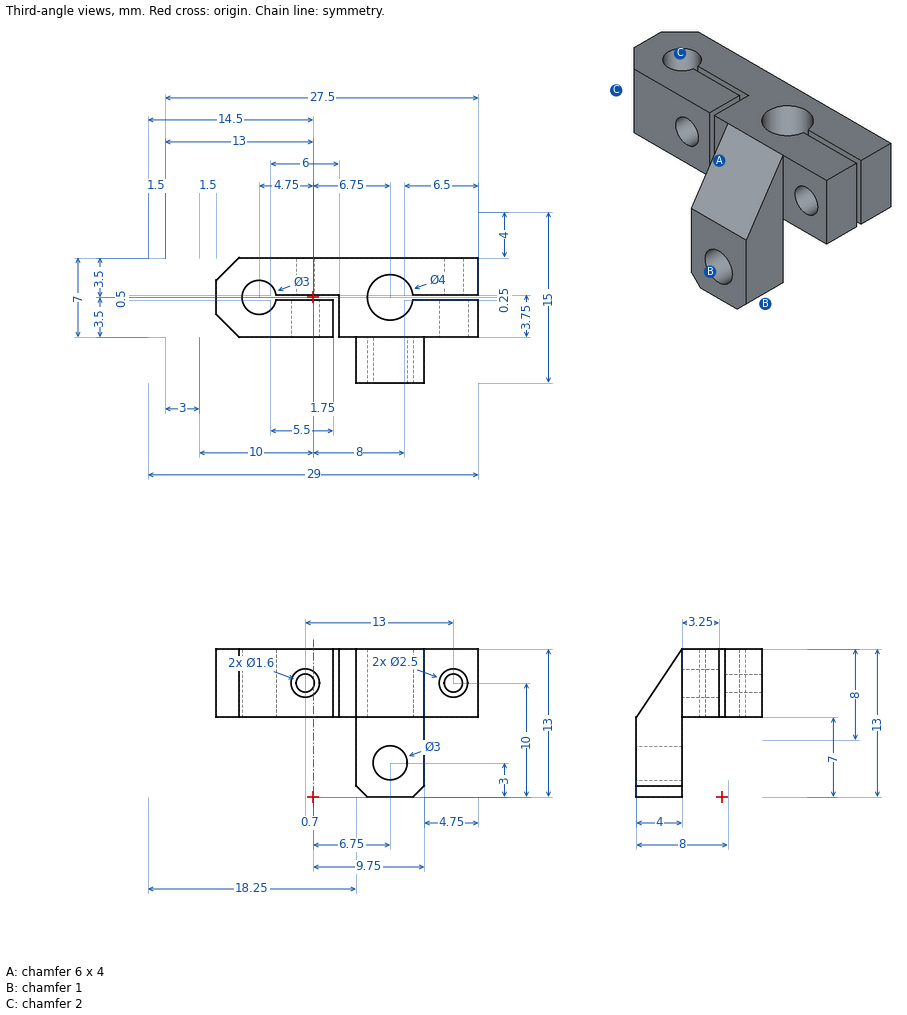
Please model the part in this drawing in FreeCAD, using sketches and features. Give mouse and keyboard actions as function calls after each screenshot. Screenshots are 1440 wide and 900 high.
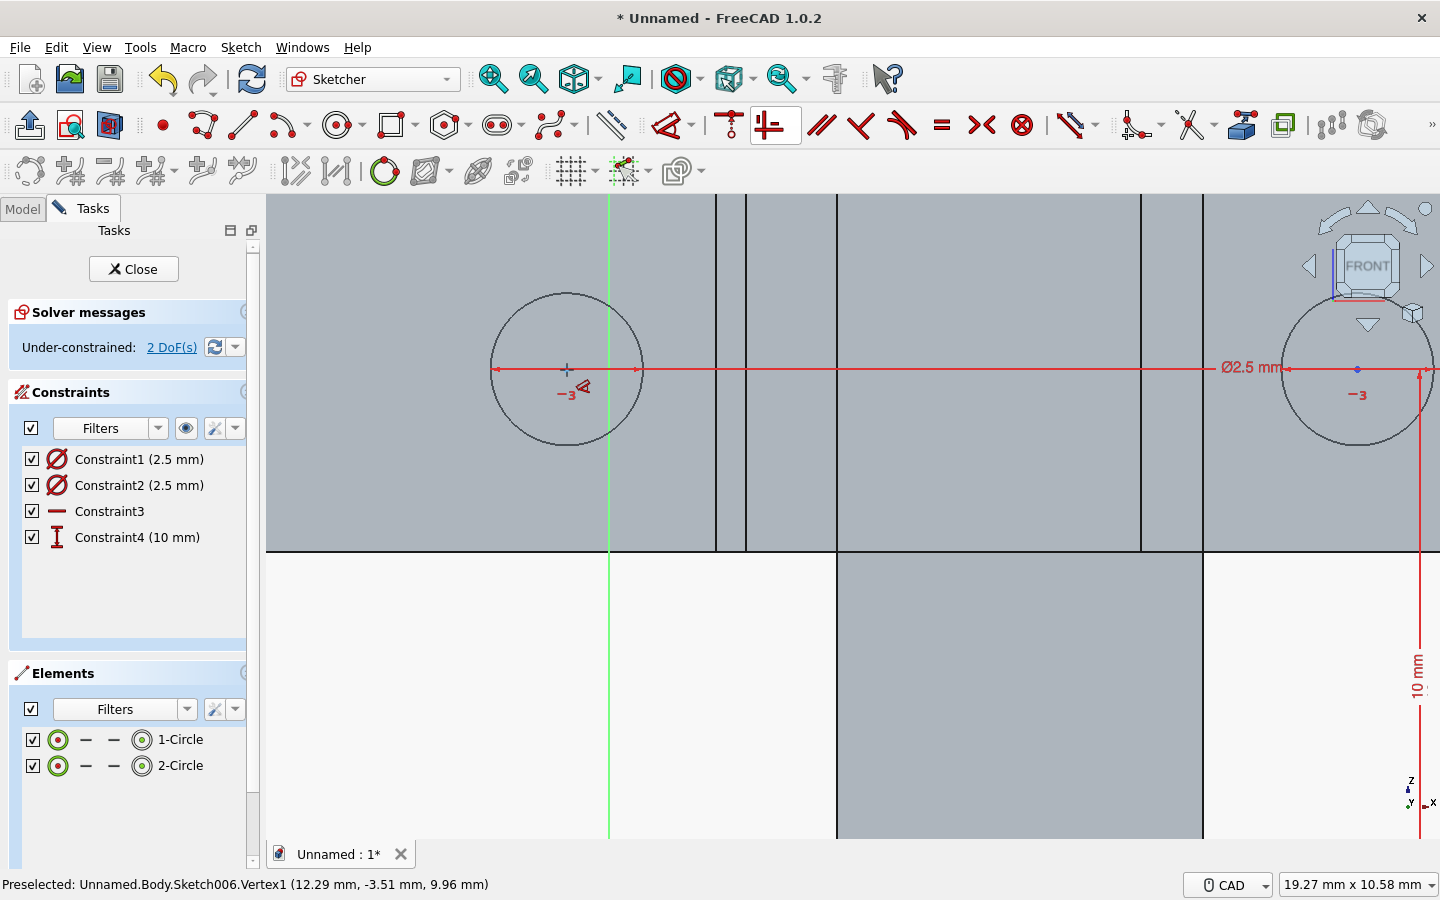
click(567, 369)
click(588, 335)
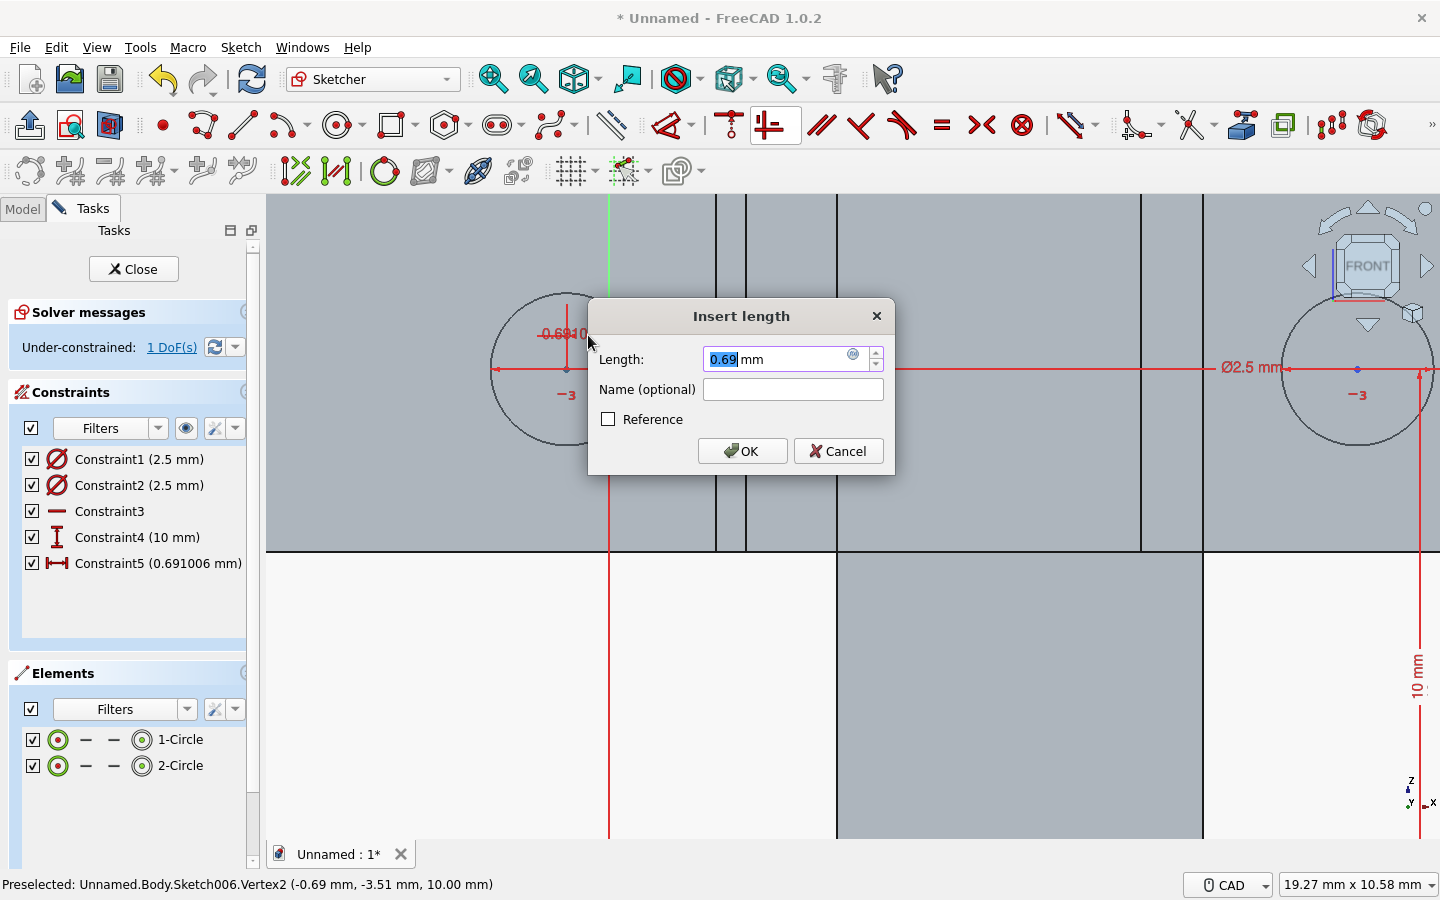
text(0.7)
key(Return)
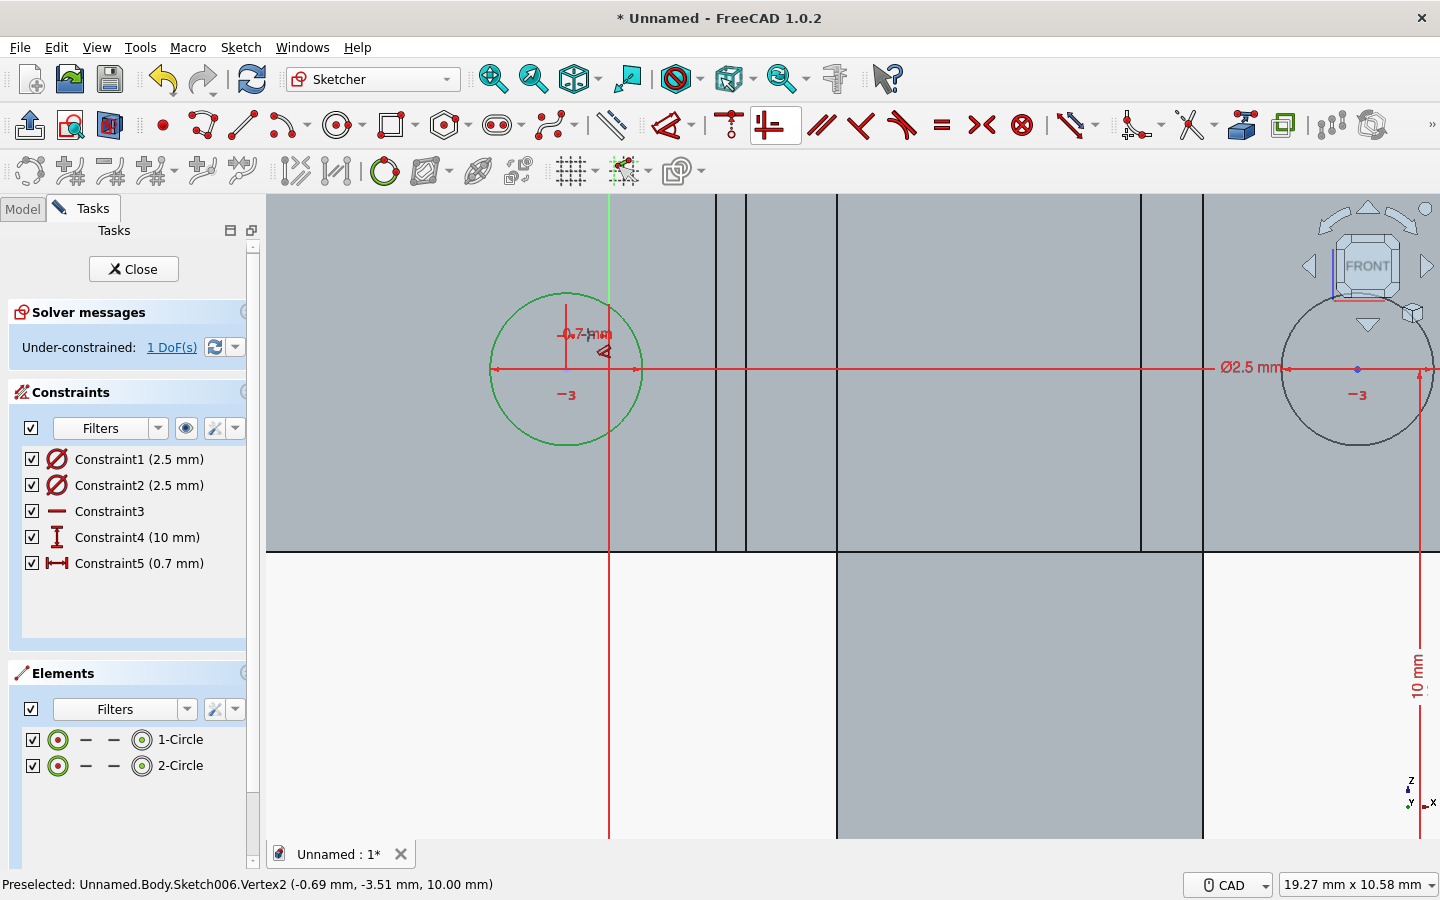
scroll(568, 371, down, 3)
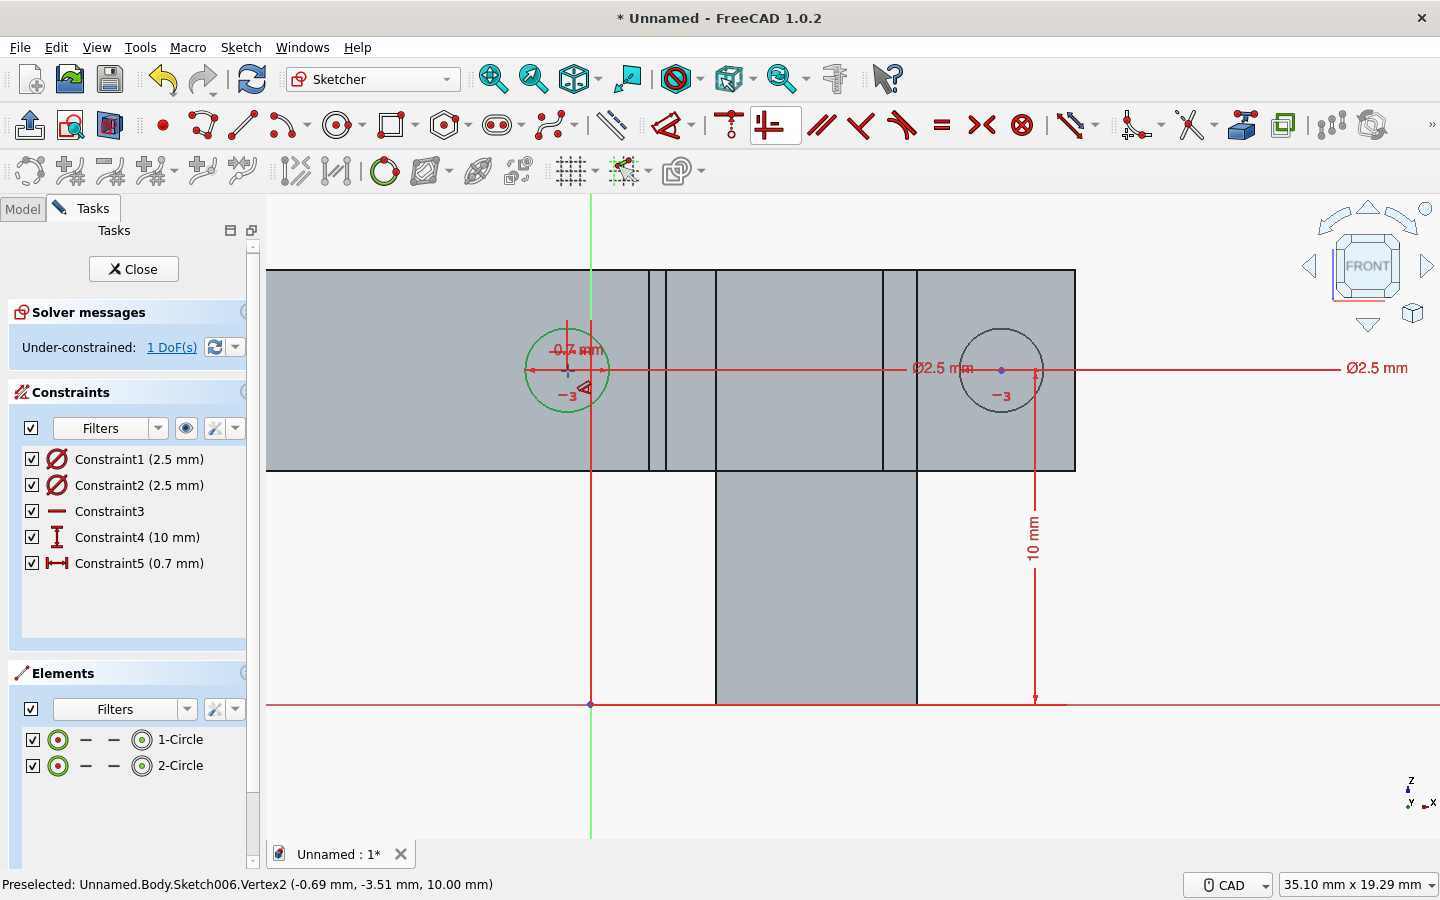
click(1001, 370)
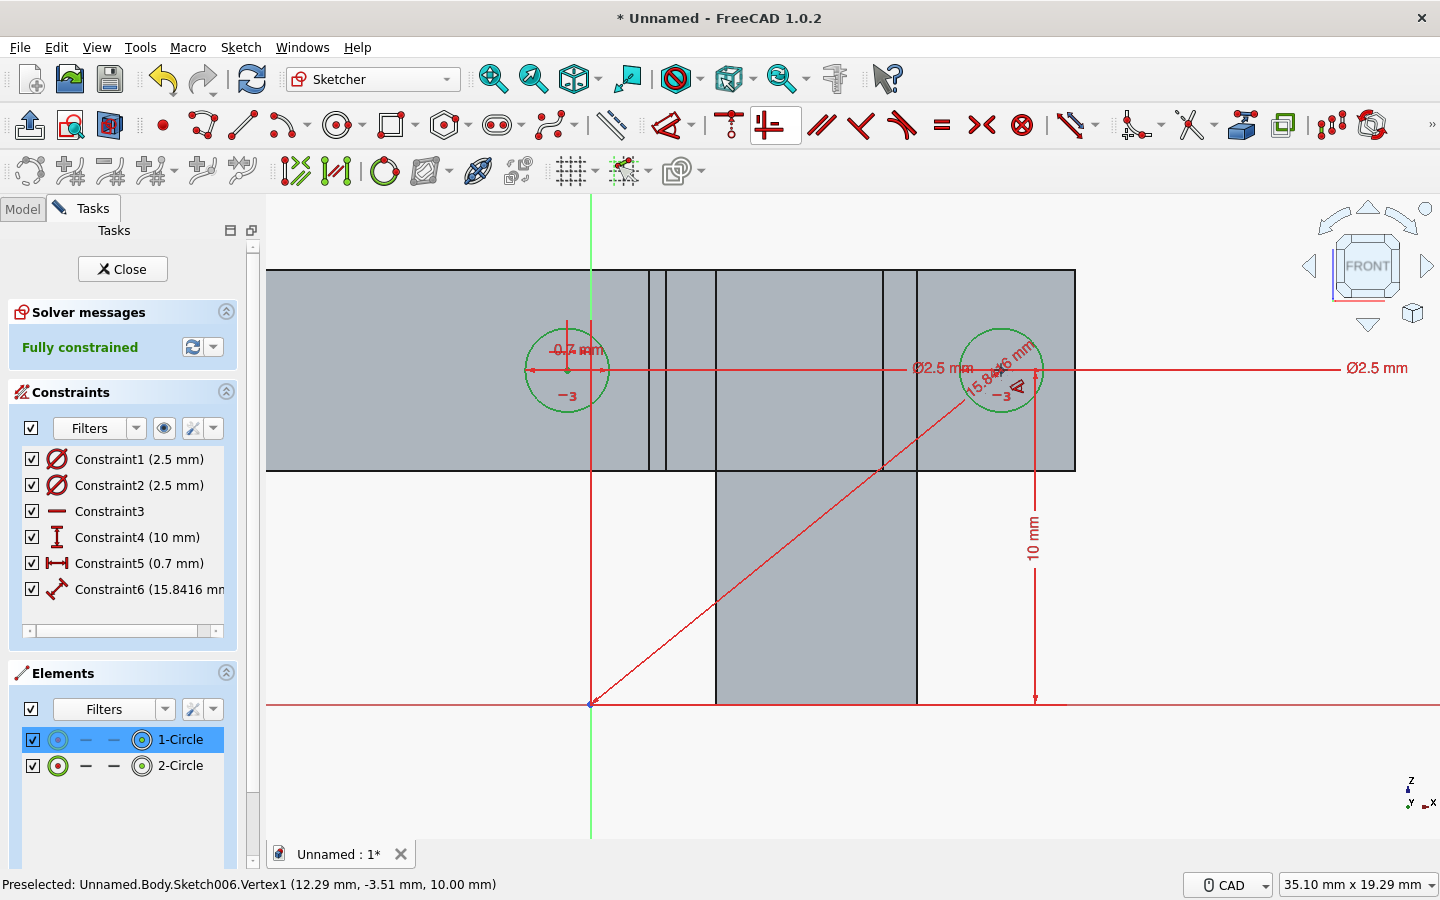
click(567, 370)
click(784, 336)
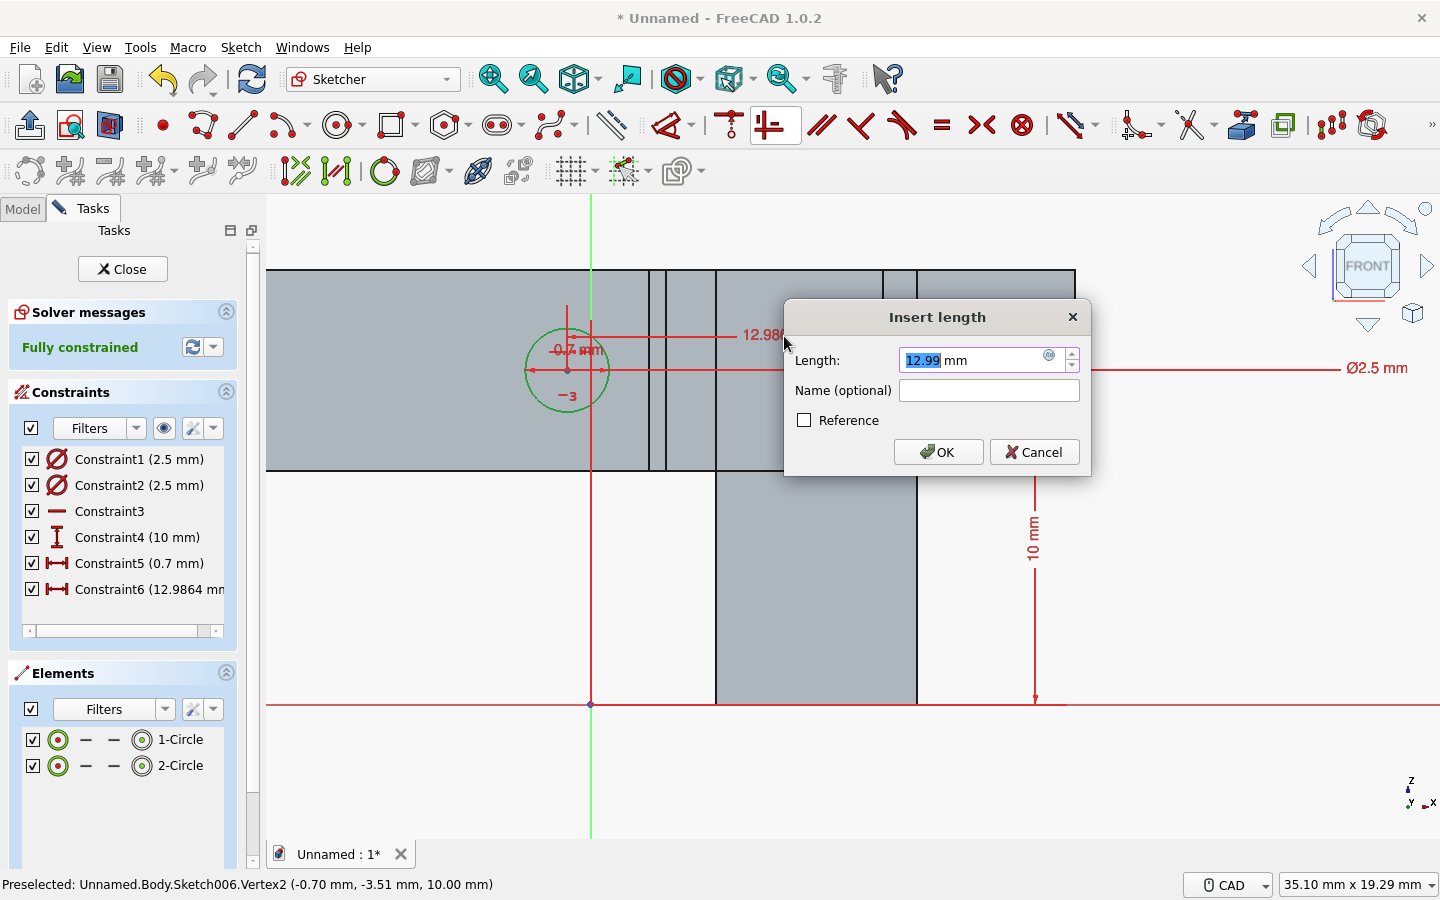
text(13)
key(Return)
key(Escape)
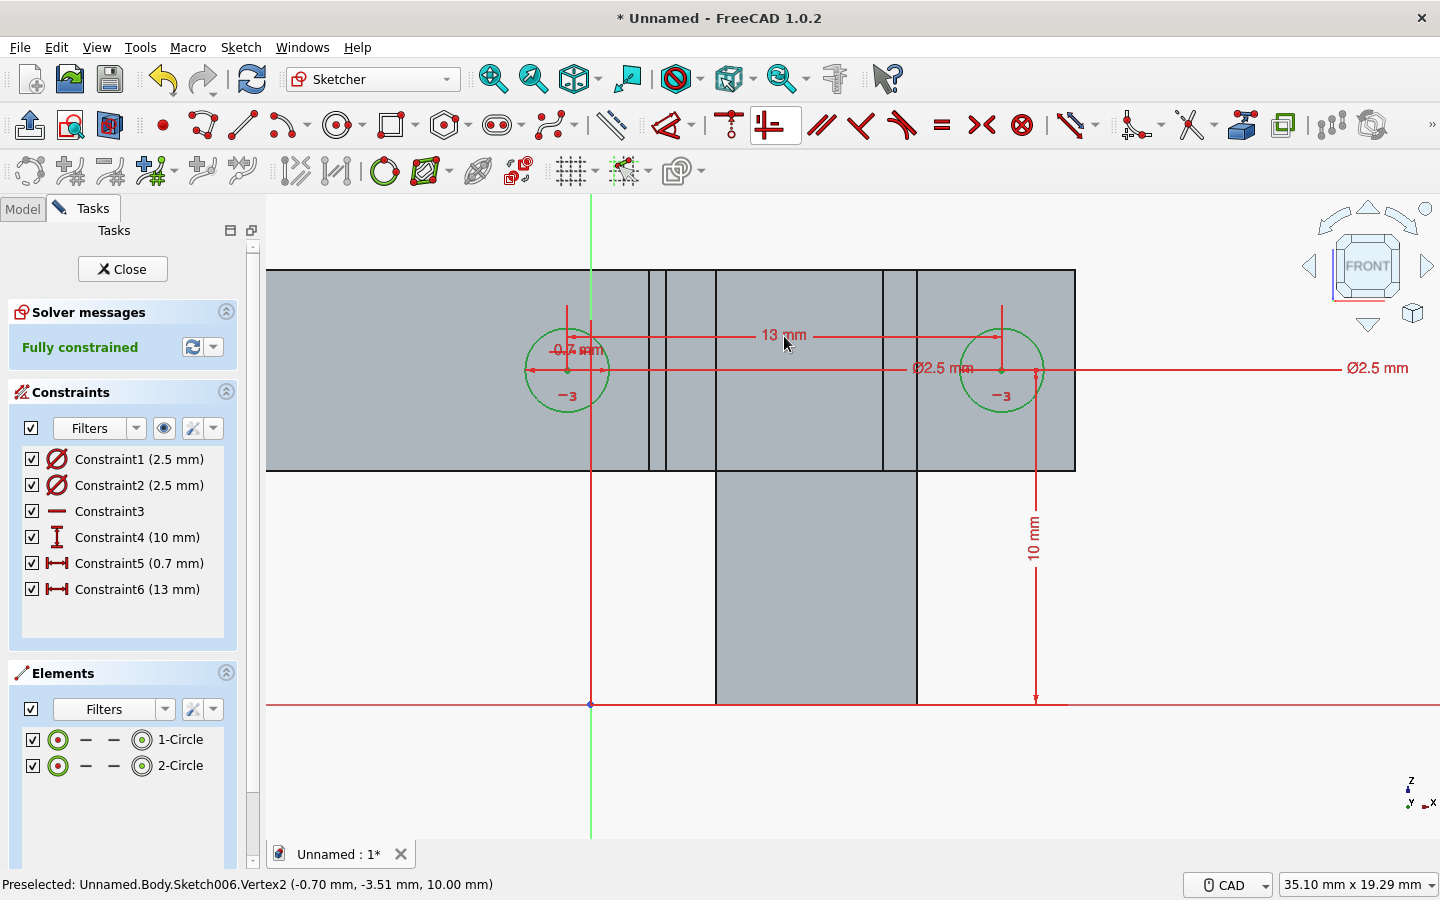
click(123, 269)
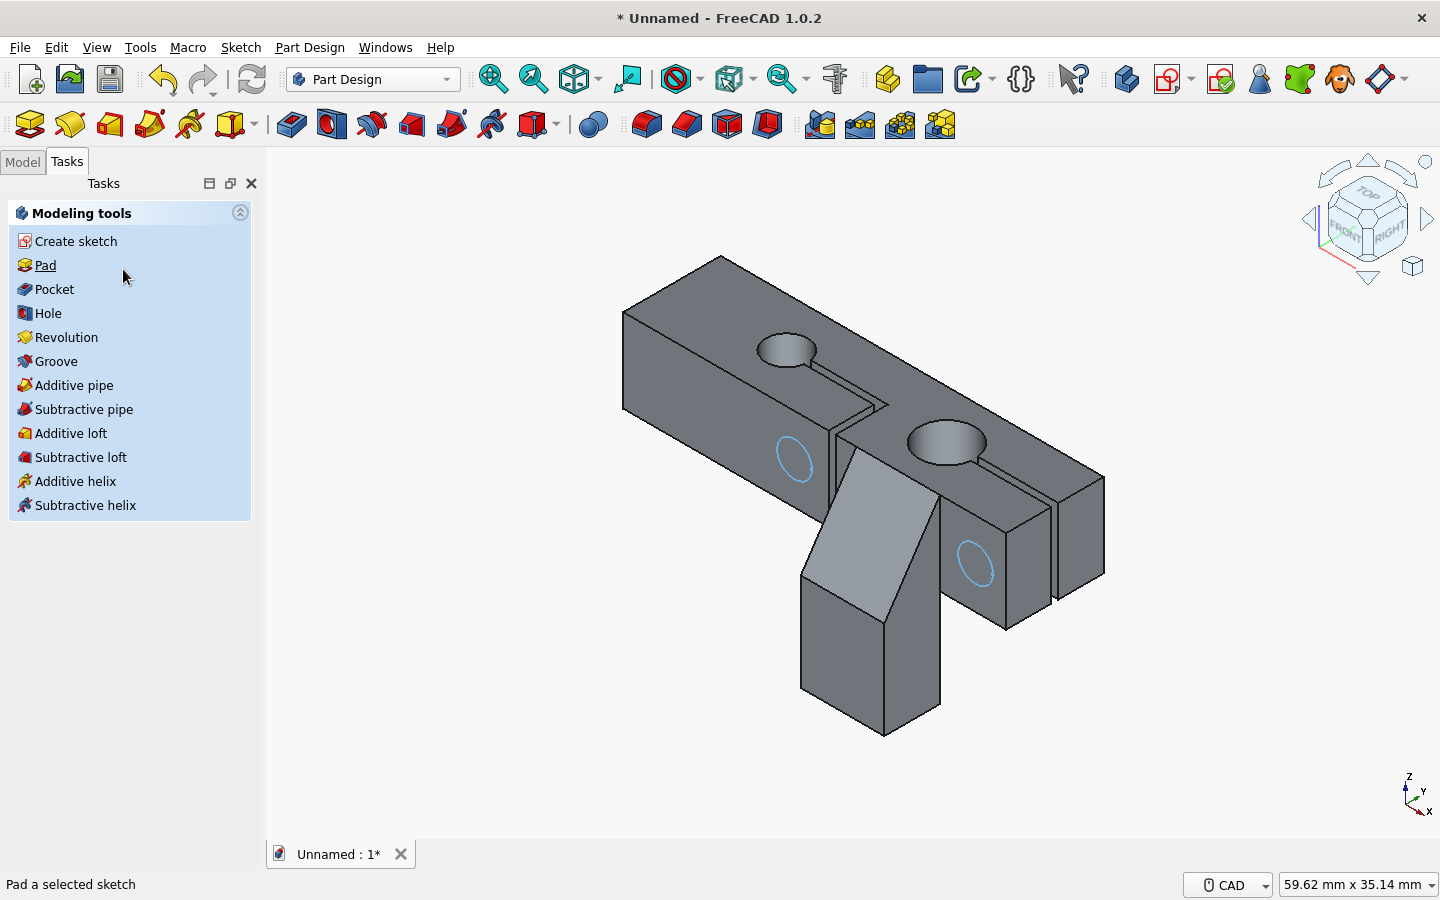
click(292, 124)